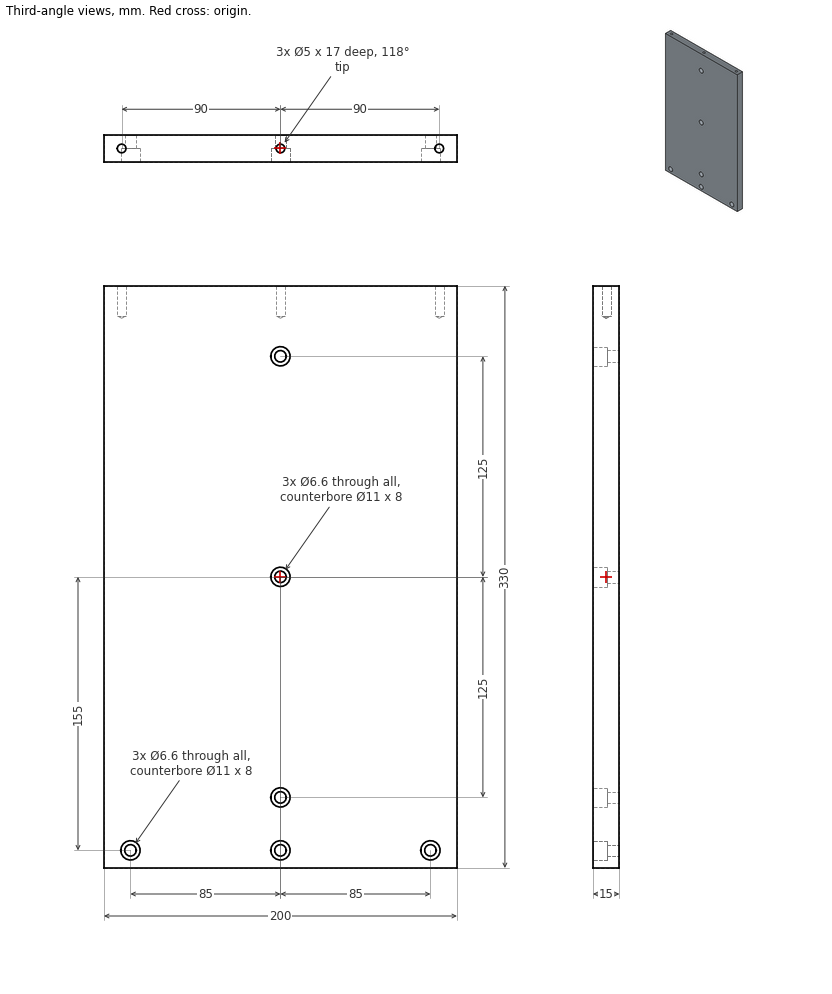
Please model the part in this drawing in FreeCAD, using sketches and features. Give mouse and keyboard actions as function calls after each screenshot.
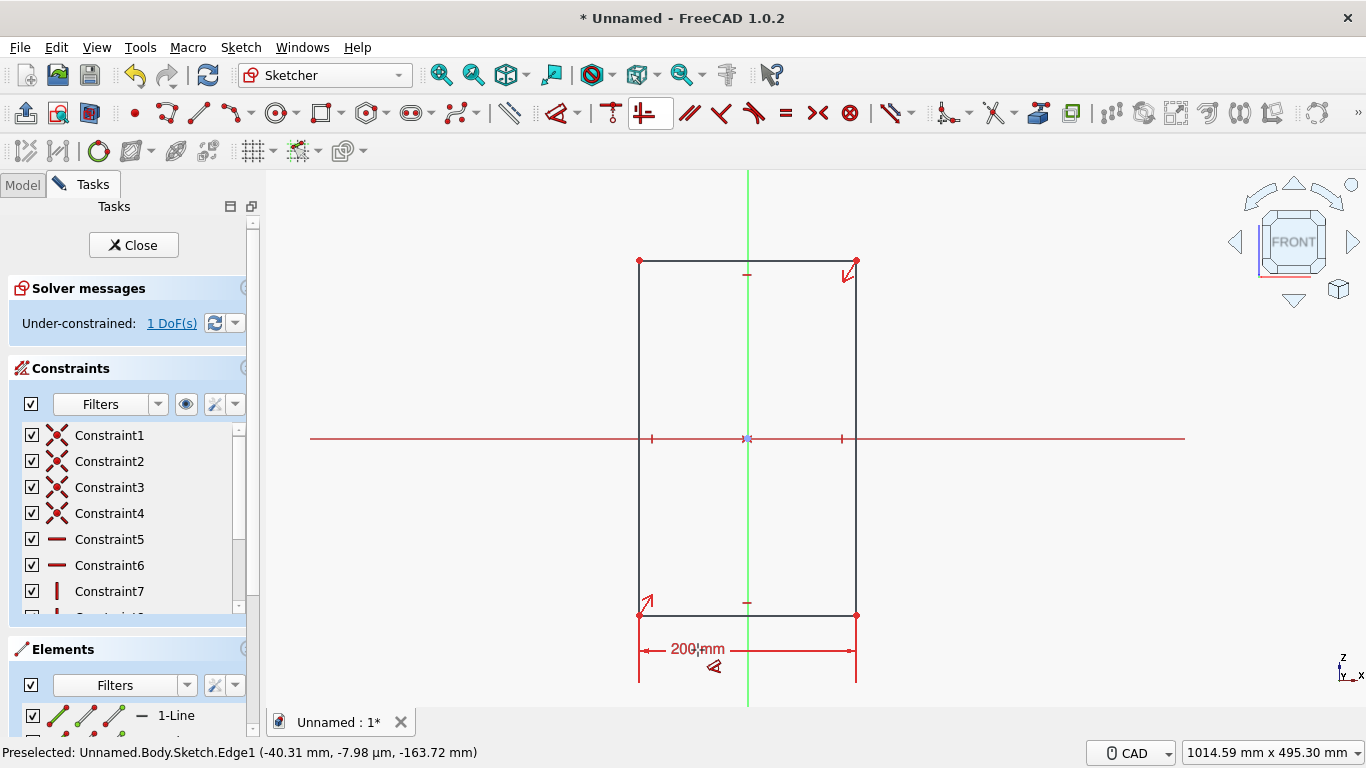
click(856, 510)
click(890, 357)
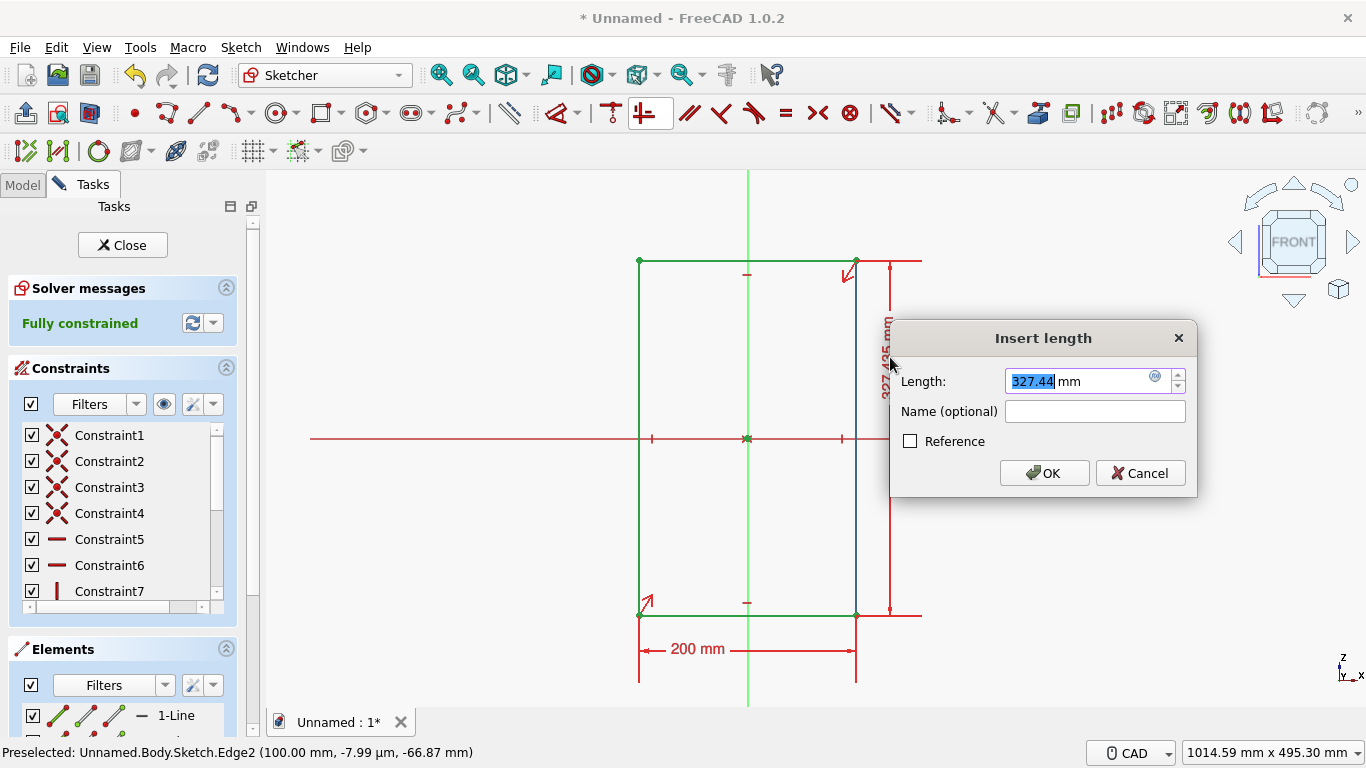
text(330)
key(Return)
key(Escape)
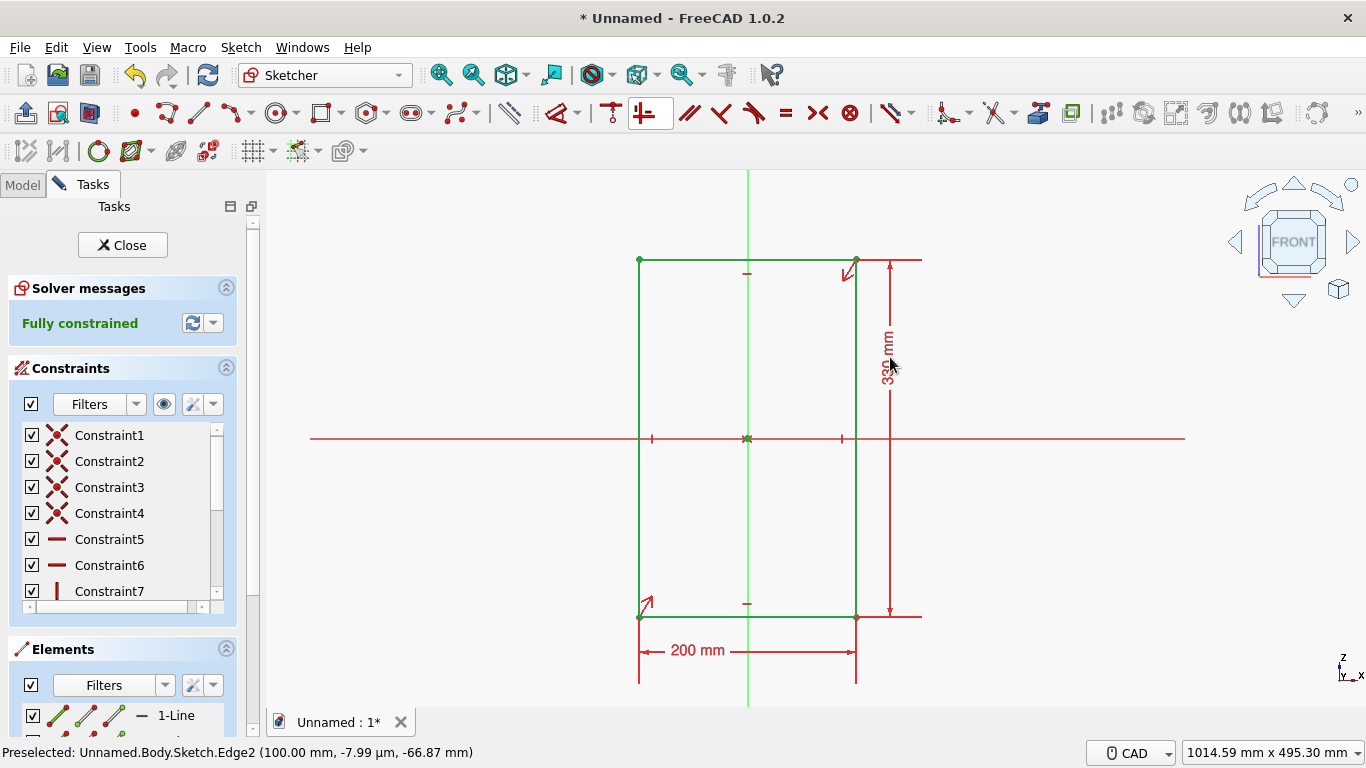
click(123, 245)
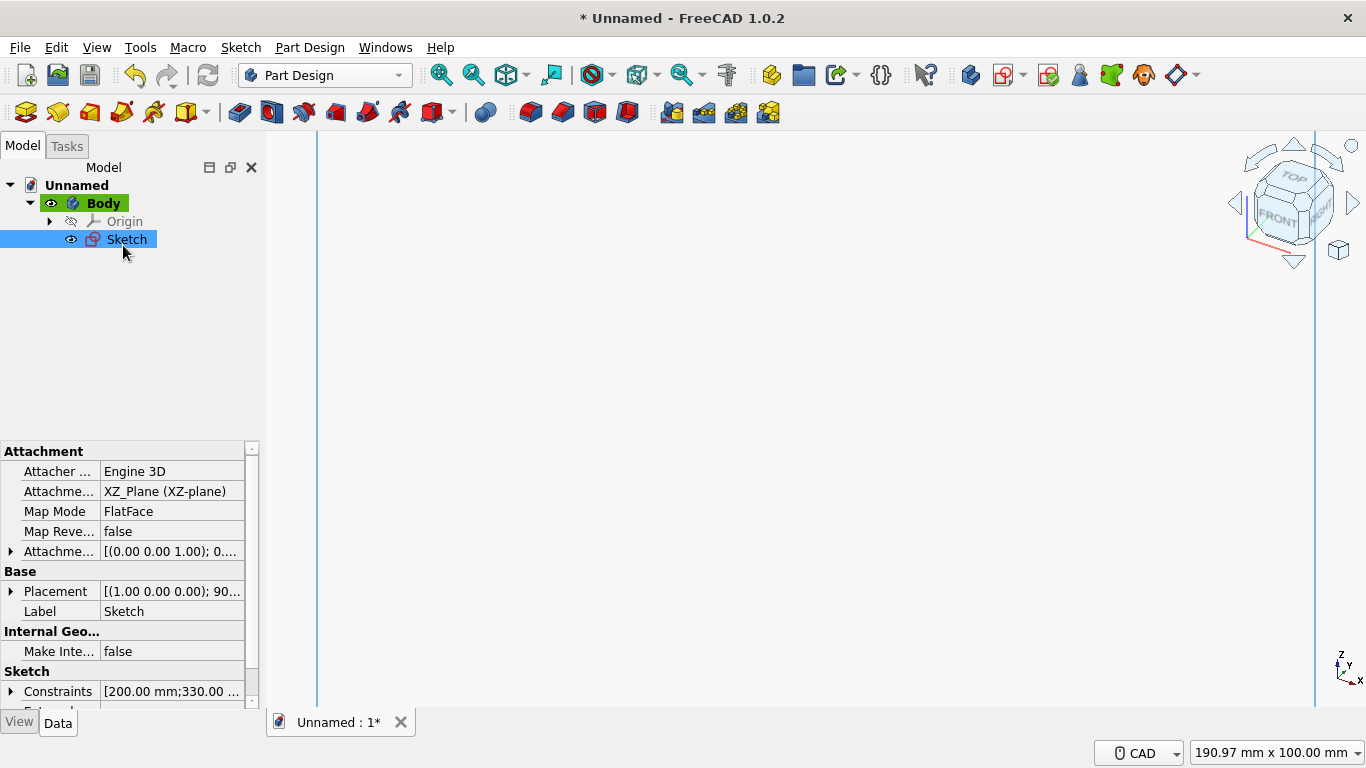
click(26, 112)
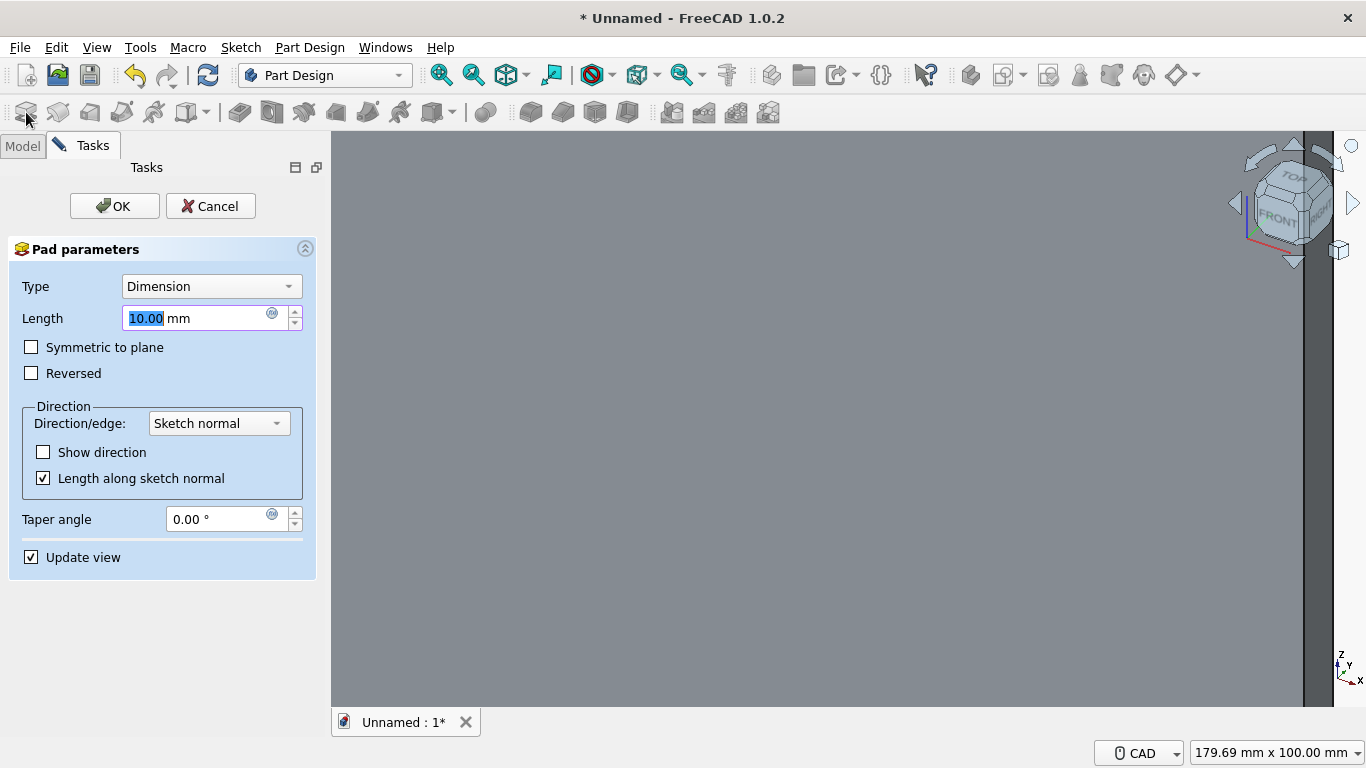
text(15)
key(Tab)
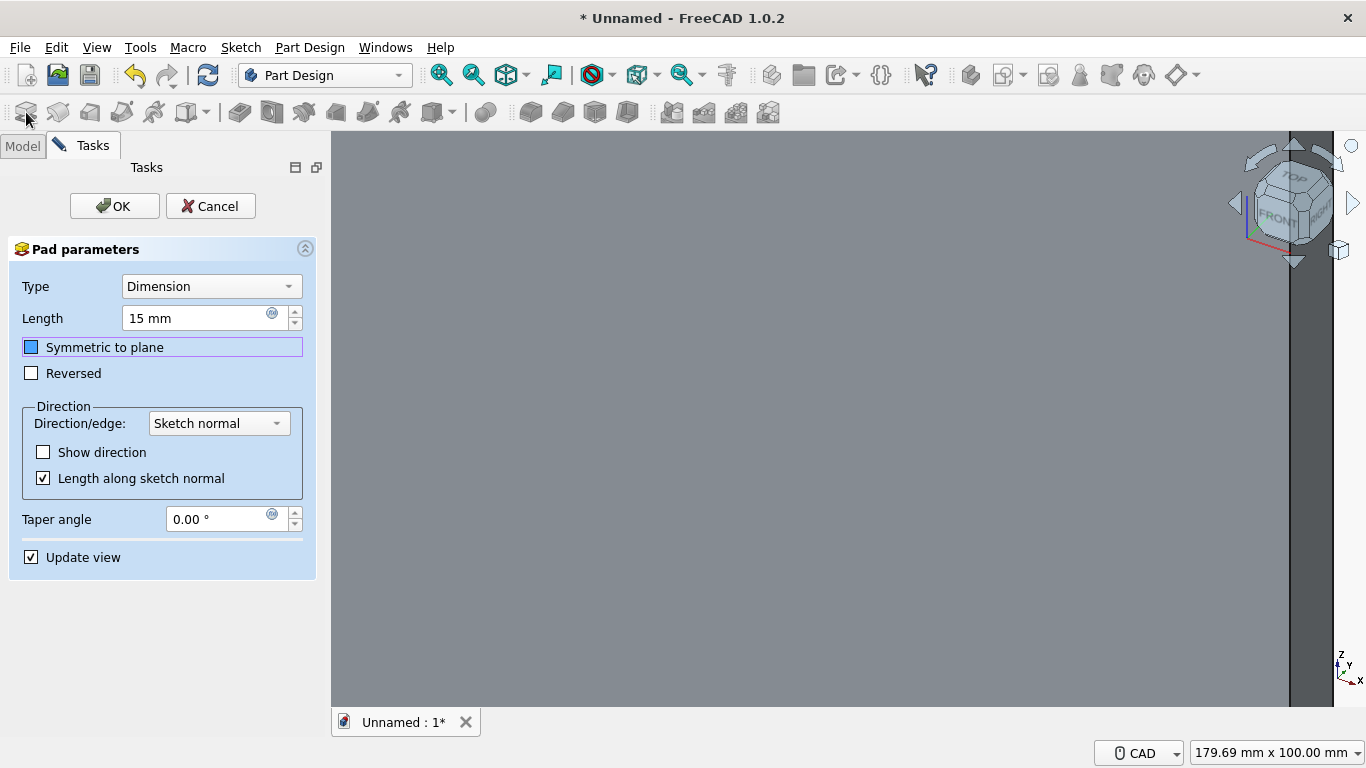
click(30, 347)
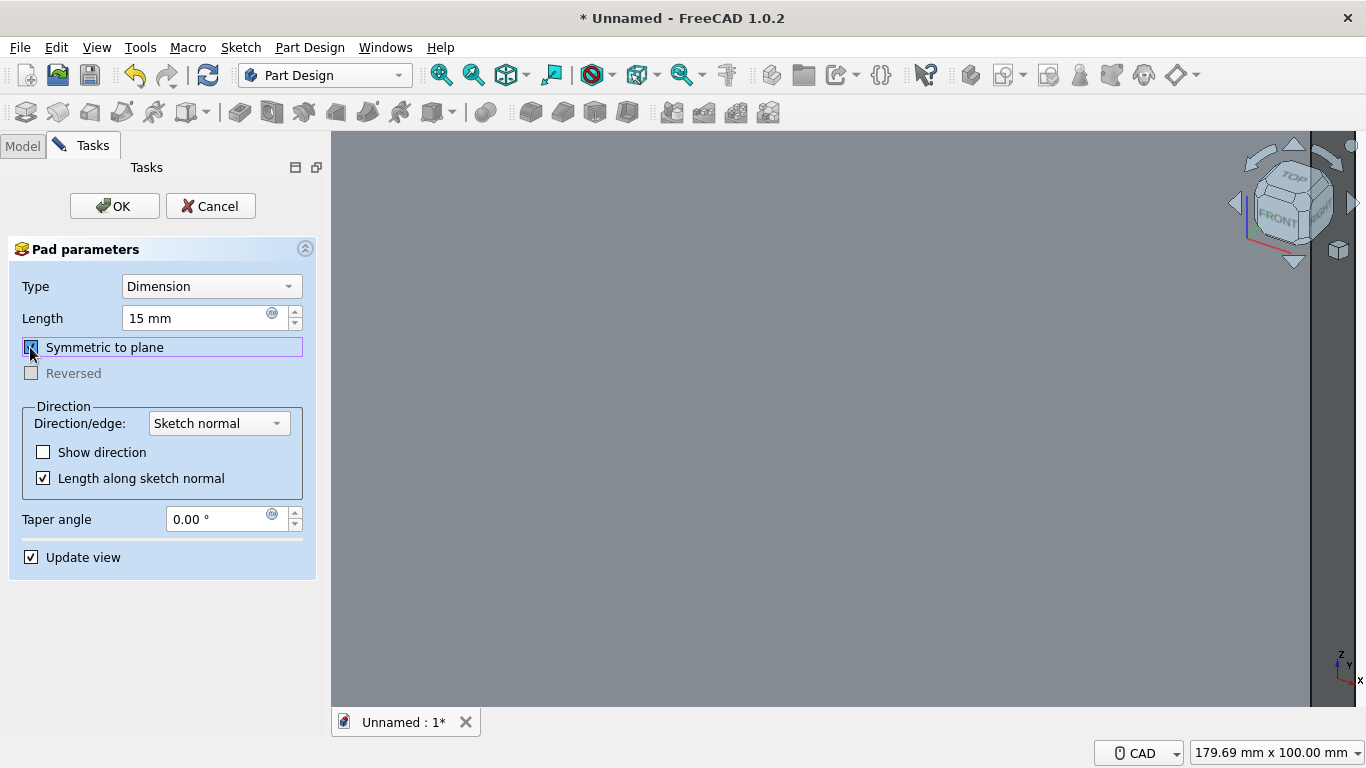
click(115, 206)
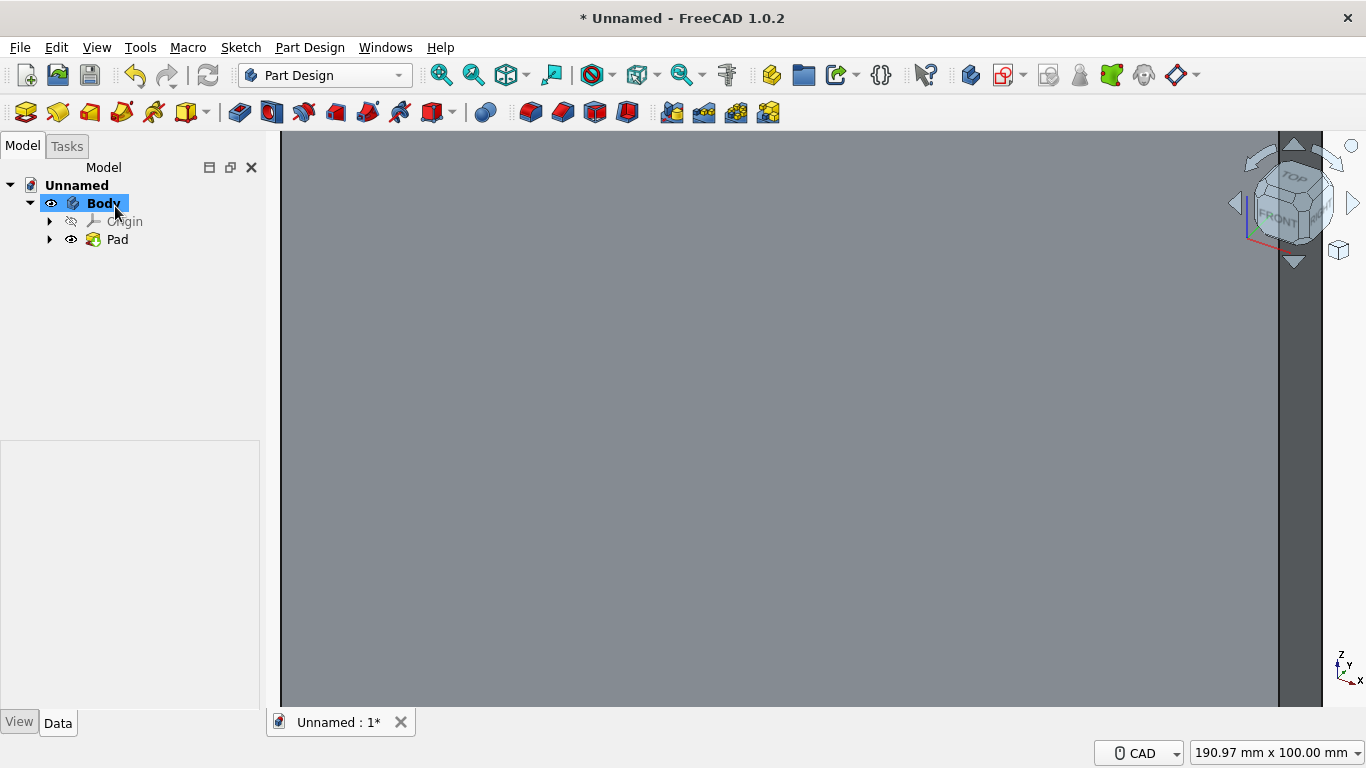
key(v)
key(f)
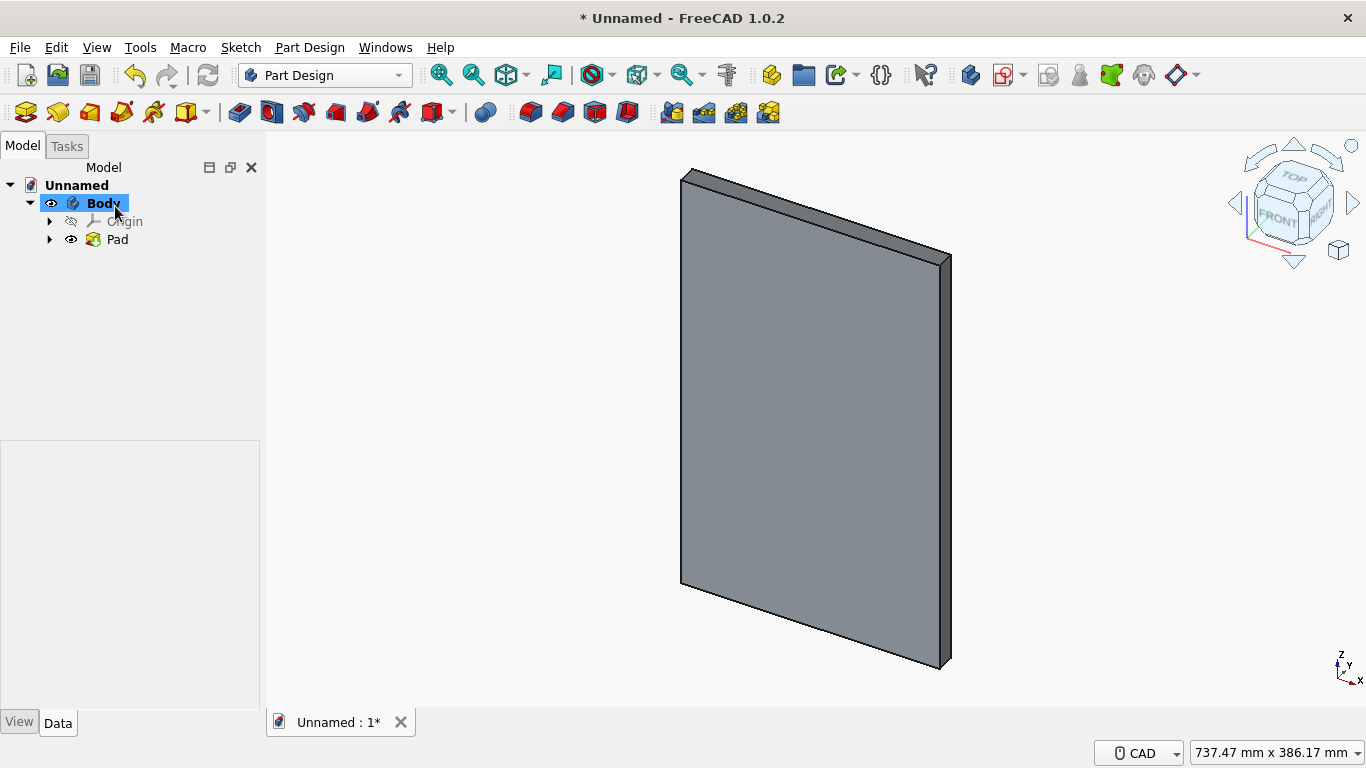
click(810, 366)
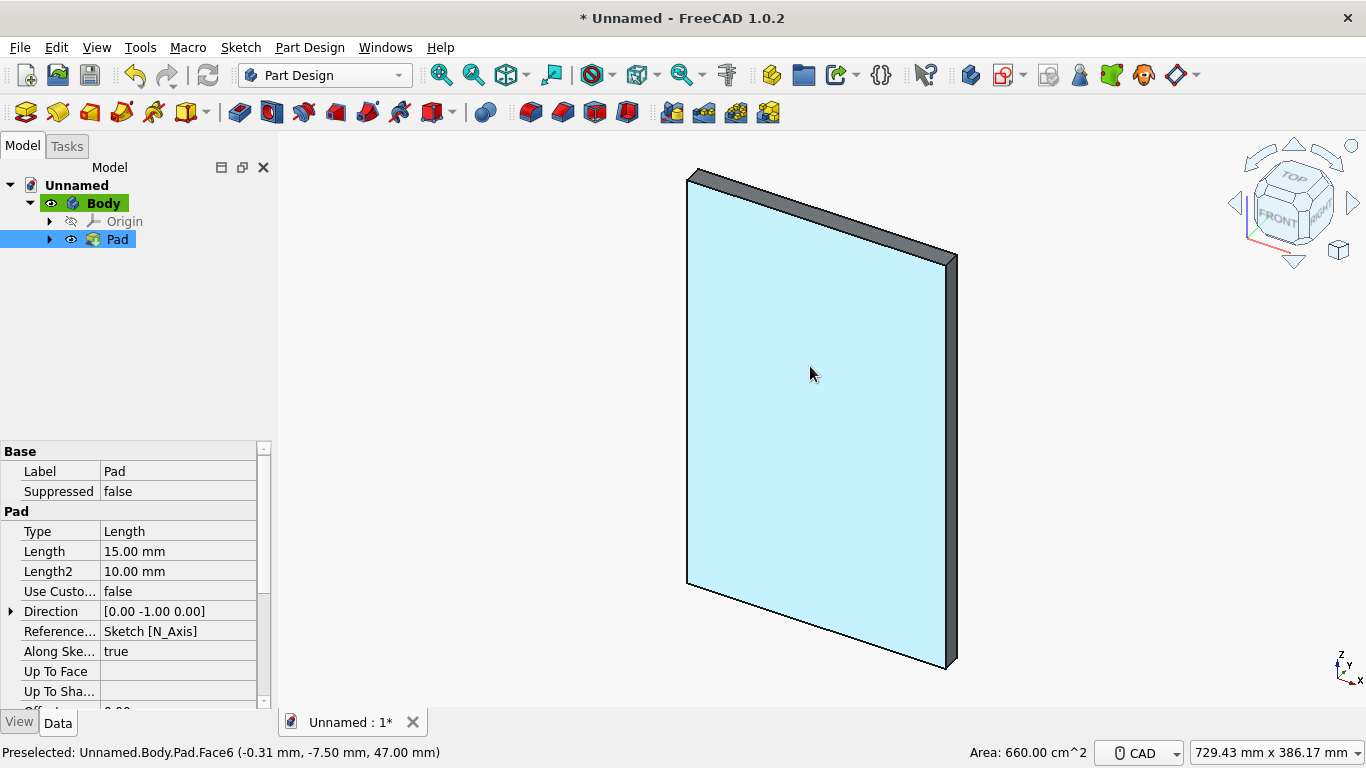
click(1004, 76)